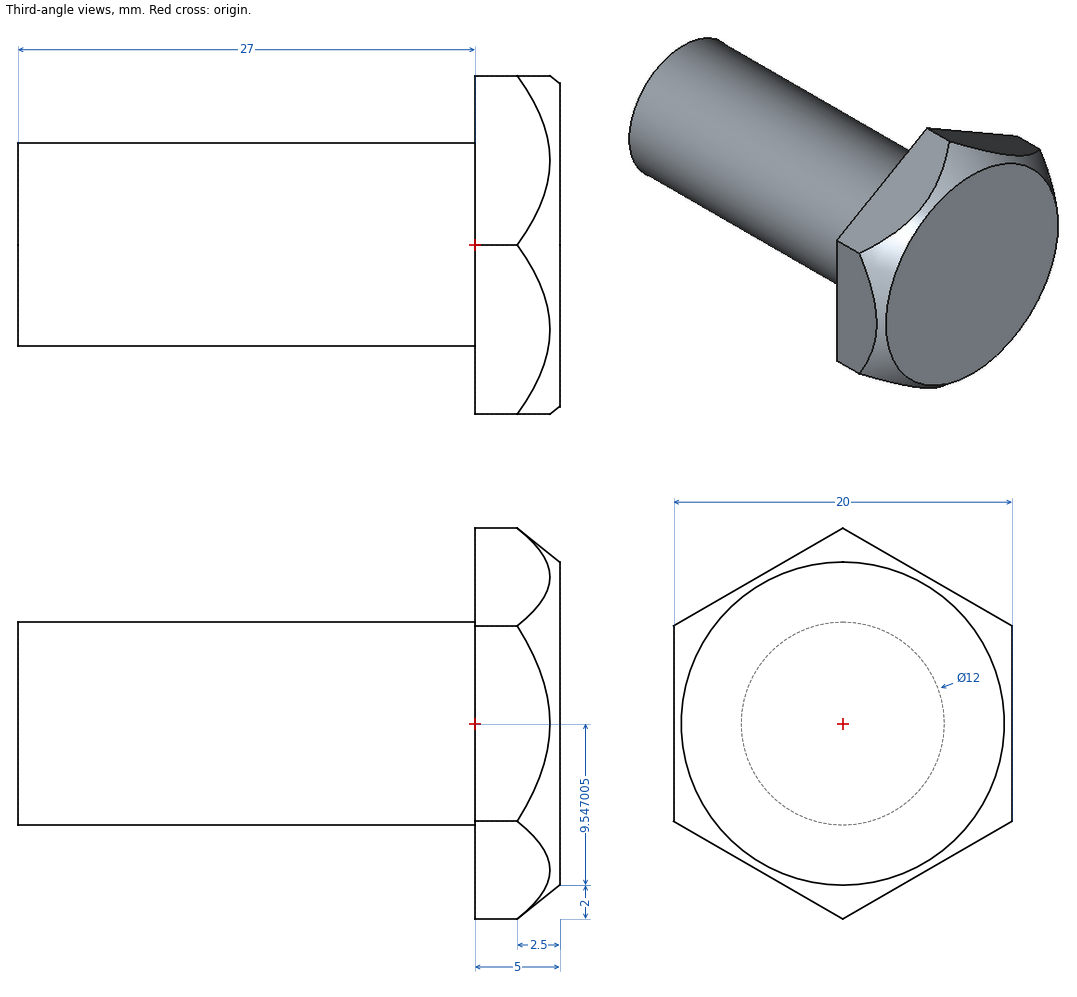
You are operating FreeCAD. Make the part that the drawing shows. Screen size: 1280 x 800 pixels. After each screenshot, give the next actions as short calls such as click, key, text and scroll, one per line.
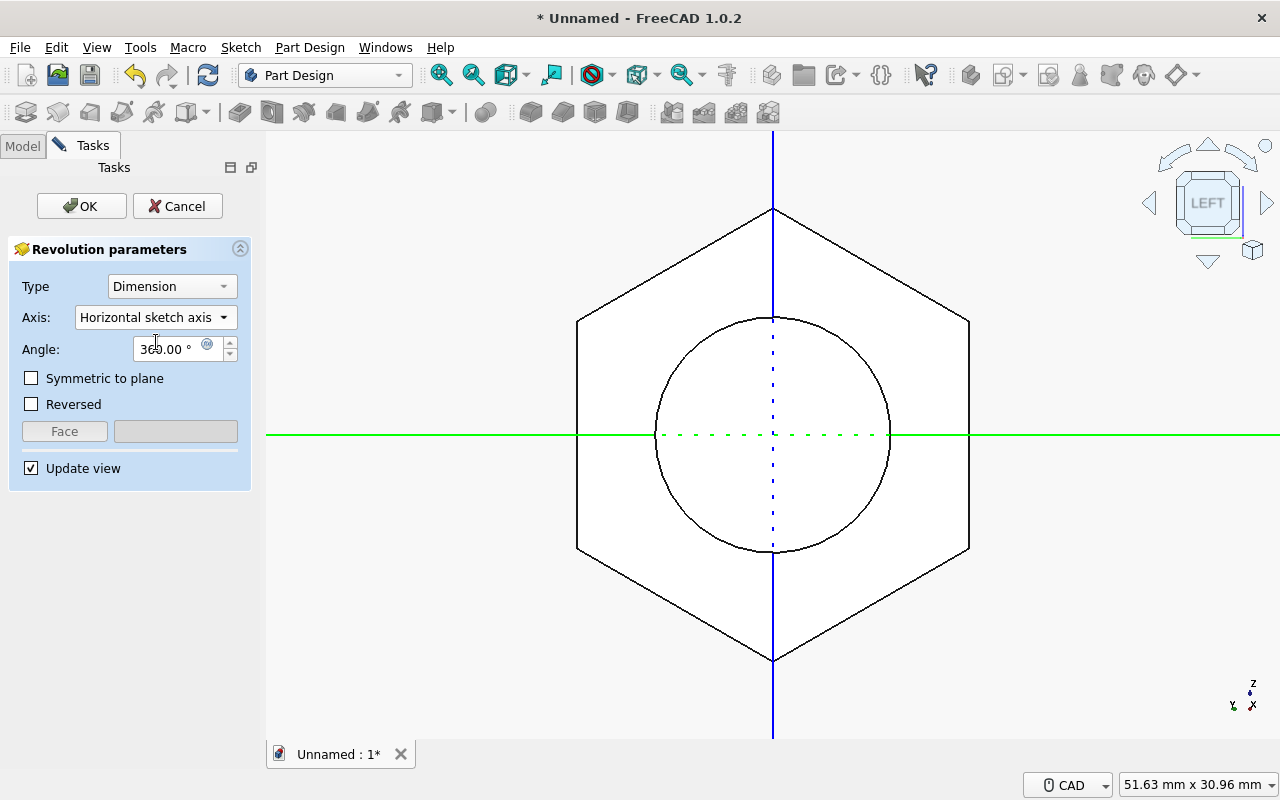
click(82, 206)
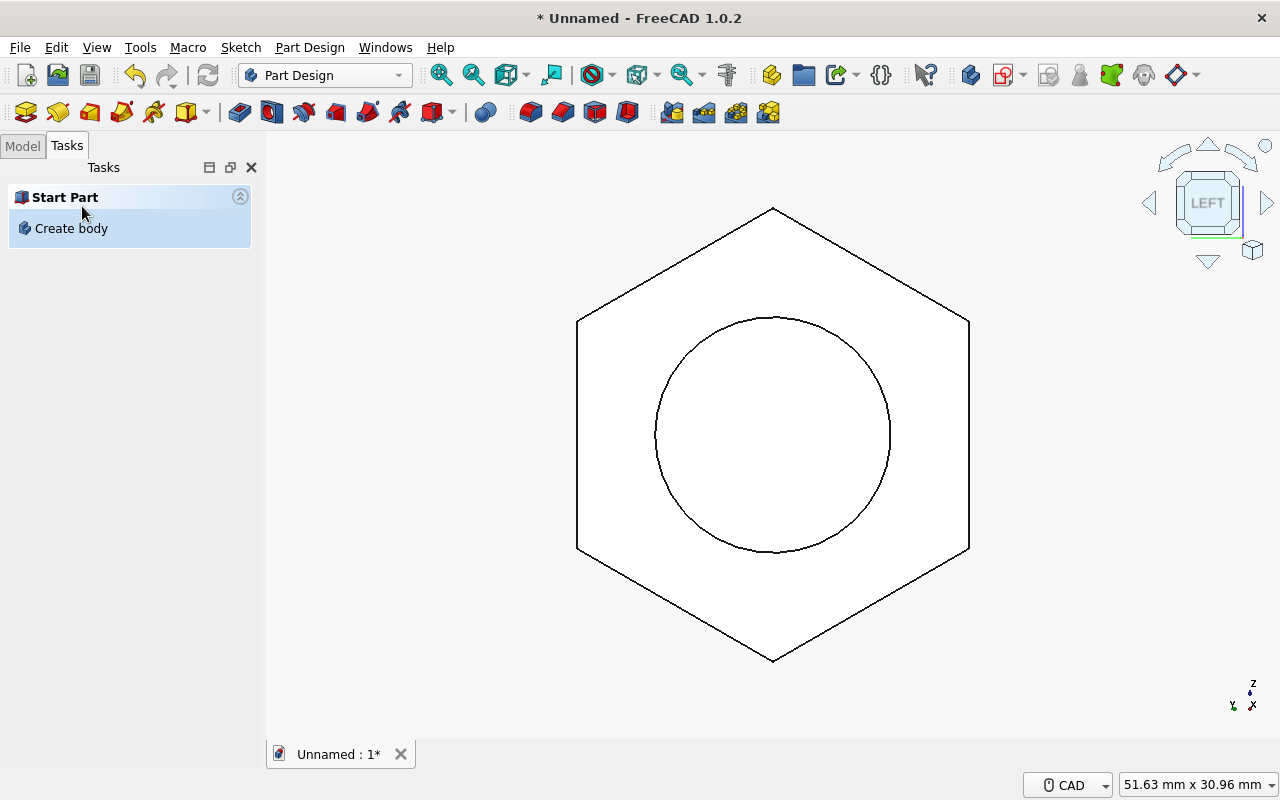
key(0)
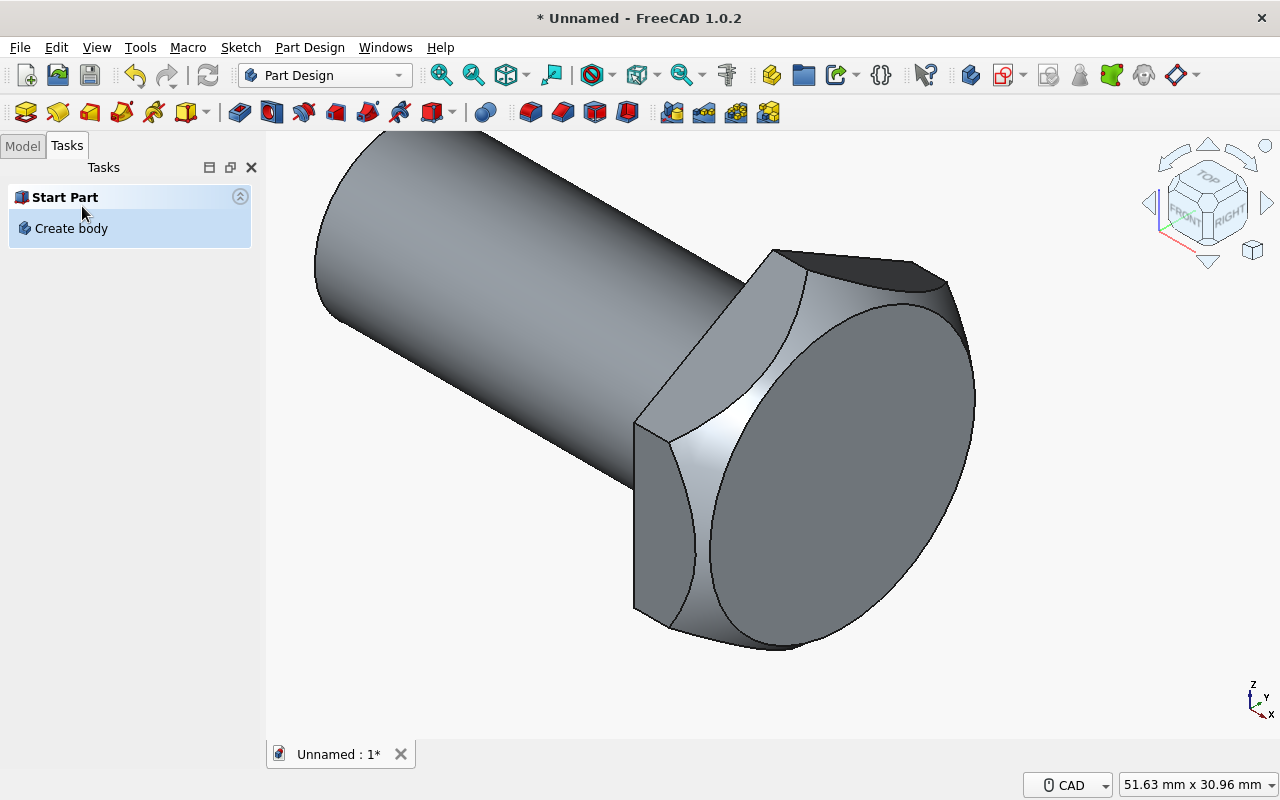
click(442, 76)